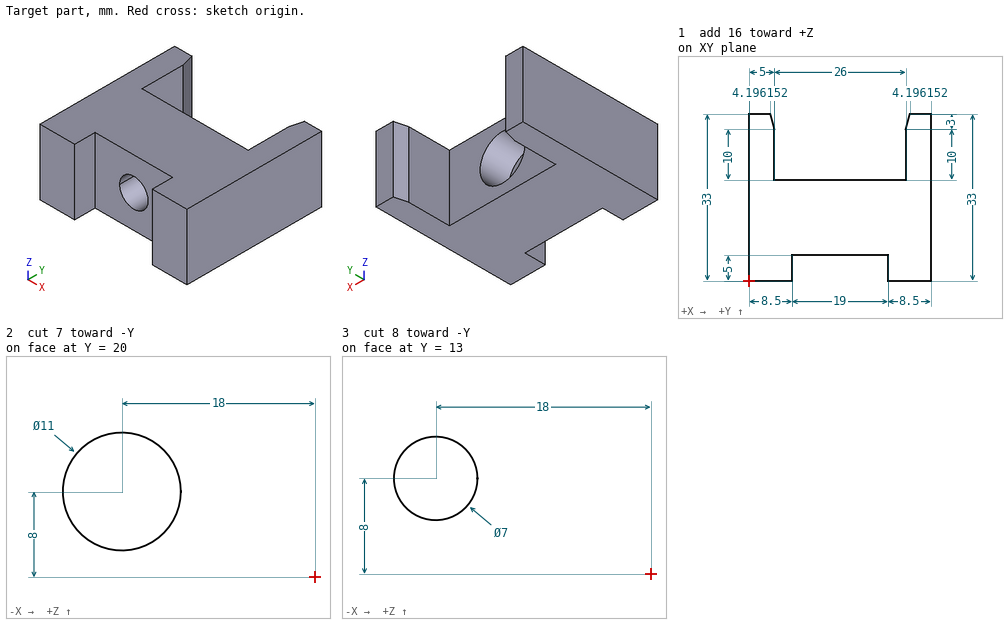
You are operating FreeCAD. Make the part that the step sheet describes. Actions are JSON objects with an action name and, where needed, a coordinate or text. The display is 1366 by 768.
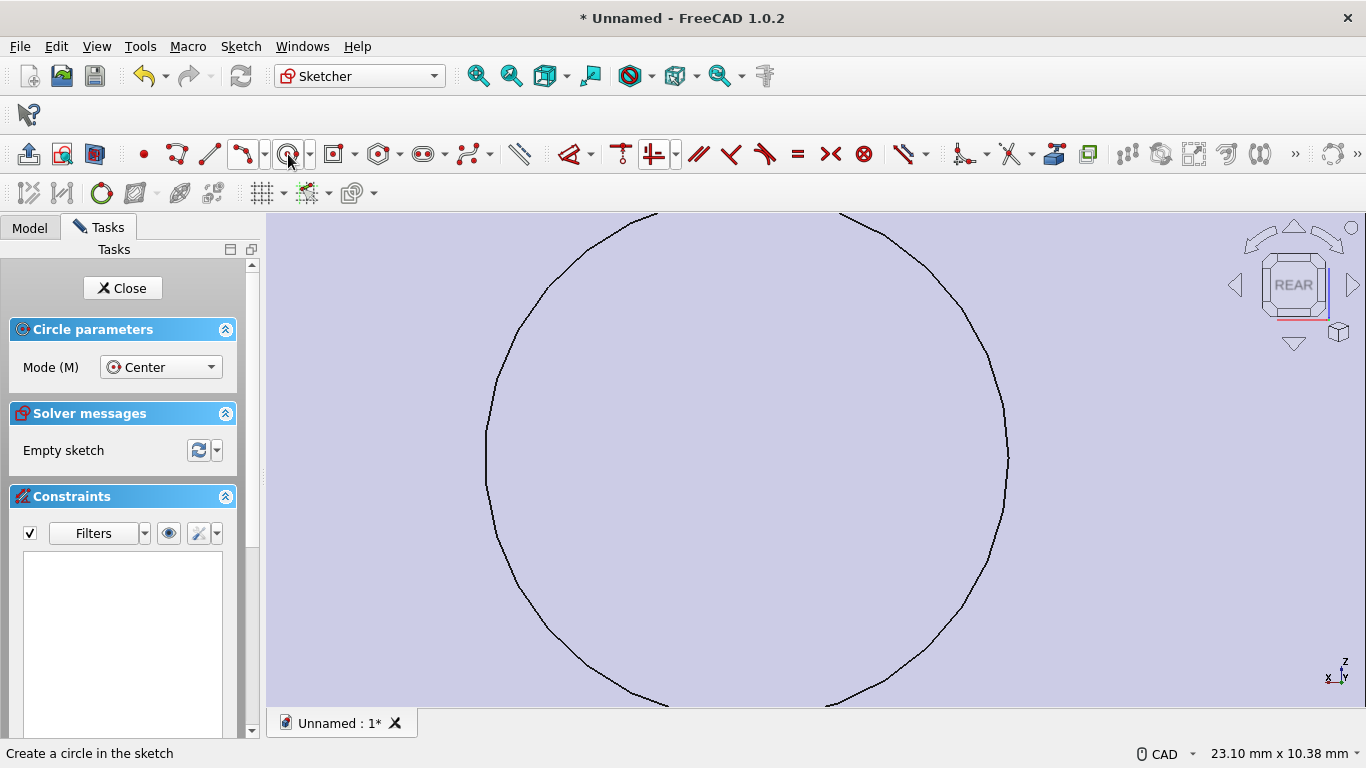
{"action": "left_click", "coordinate": [747, 458]}
{"action": "mouse_move", "coordinate": [865, 340]}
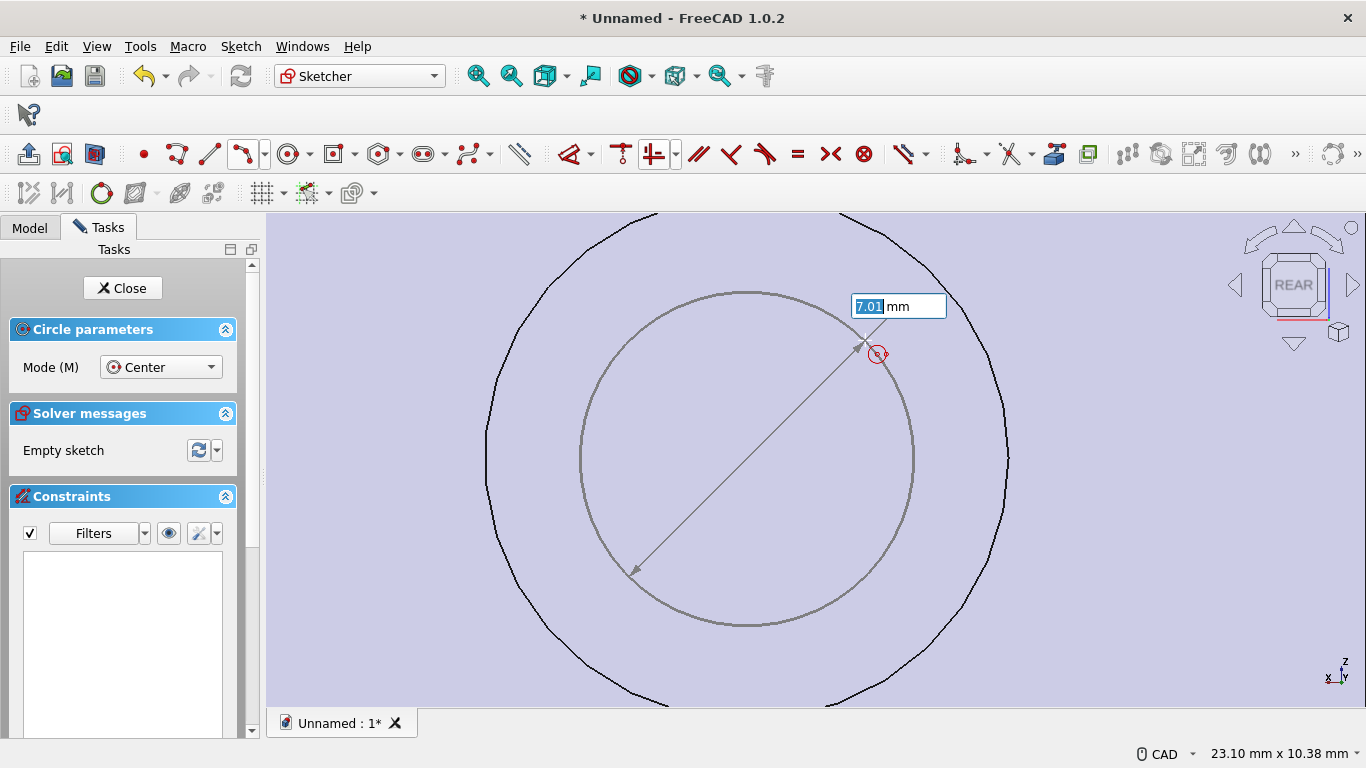
{"action": "type", "text": "7"}
{"action": "key", "text": "Return"}
{"action": "key", "text": "Escape"}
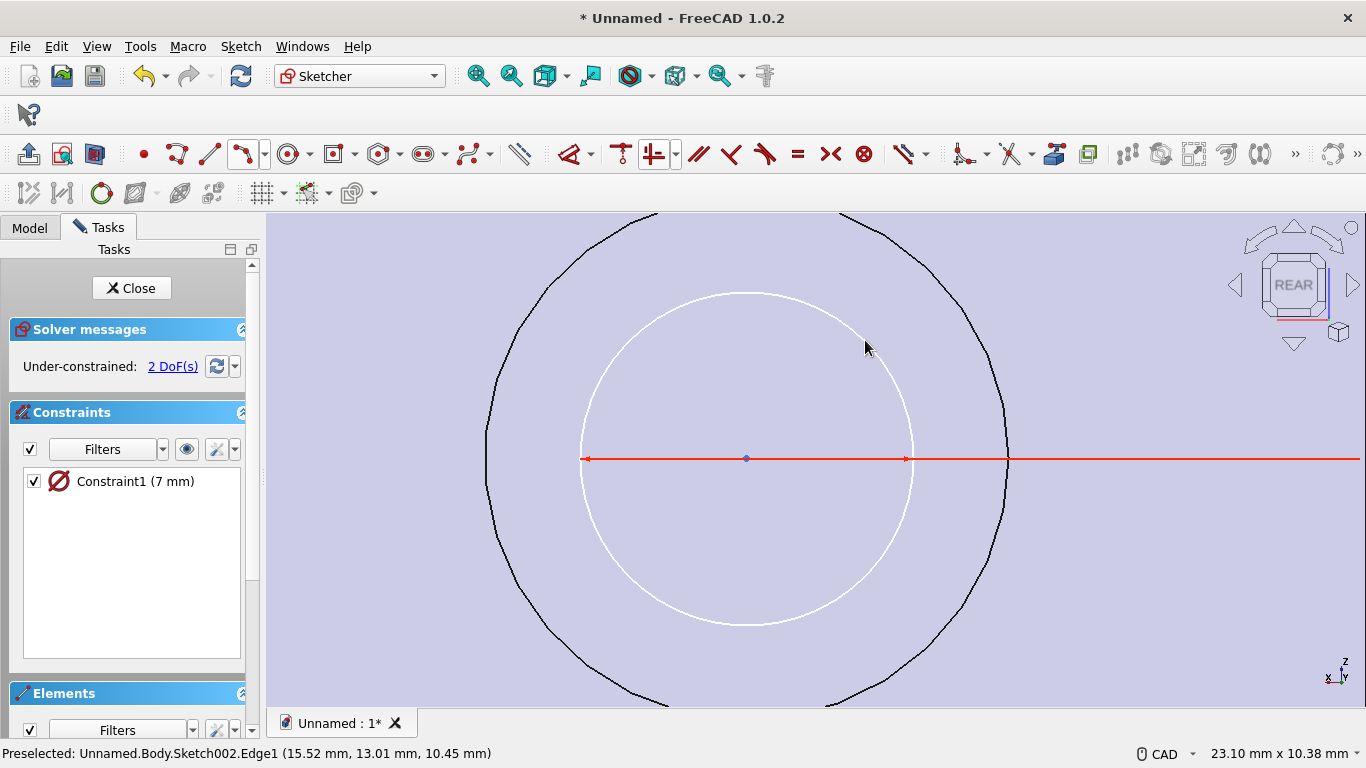
{"action": "left_click", "coordinate": [568, 154]}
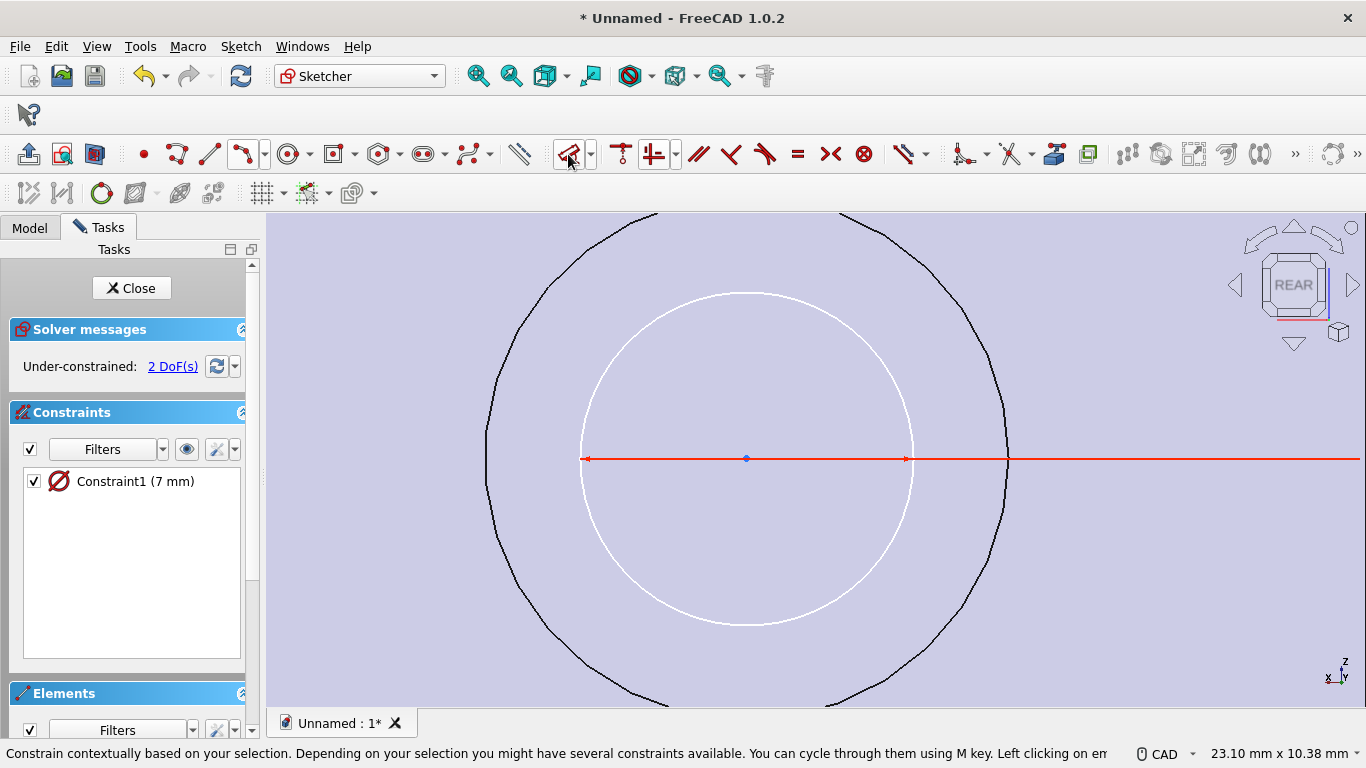
{"action": "left_click", "coordinate": [747, 459]}
{"action": "left_click", "coordinate": [713, 569]}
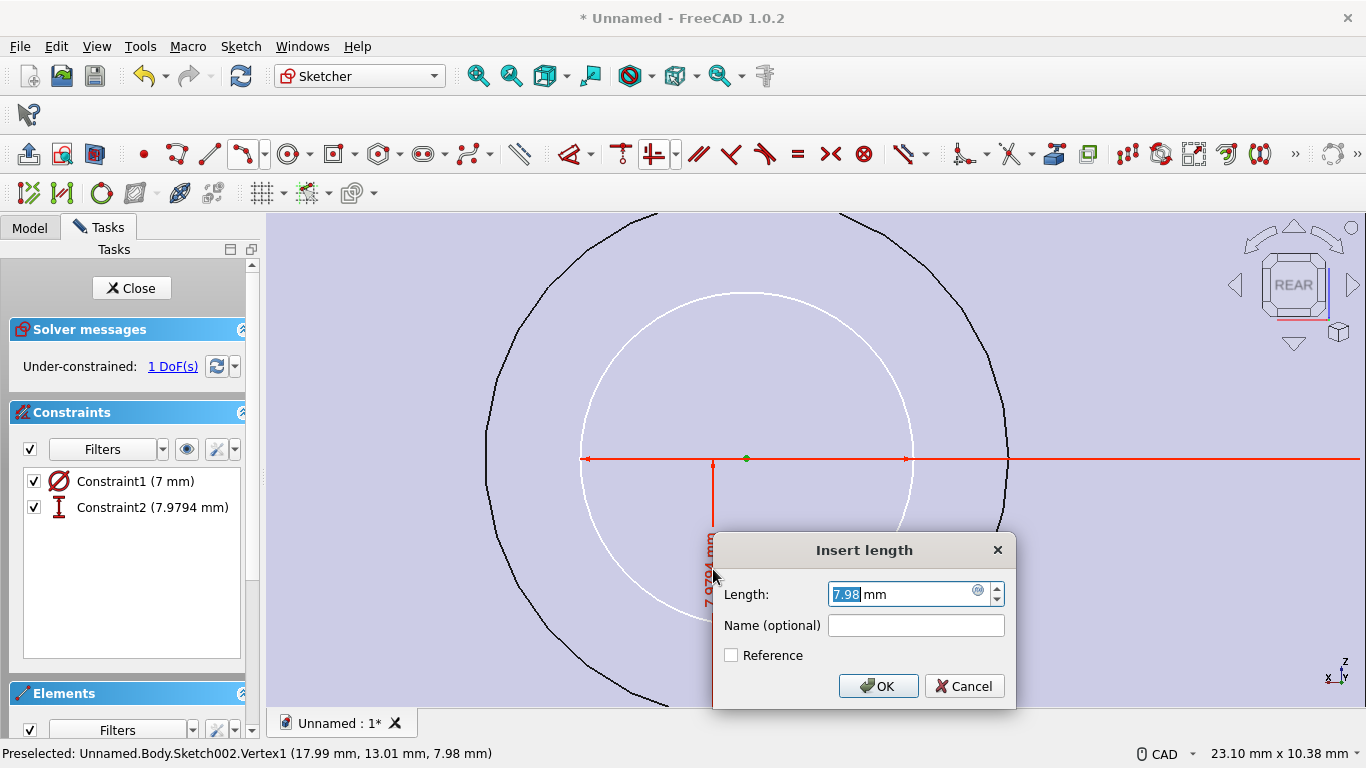
{"action": "type", "text": "8"}
{"action": "key", "text": "Return"}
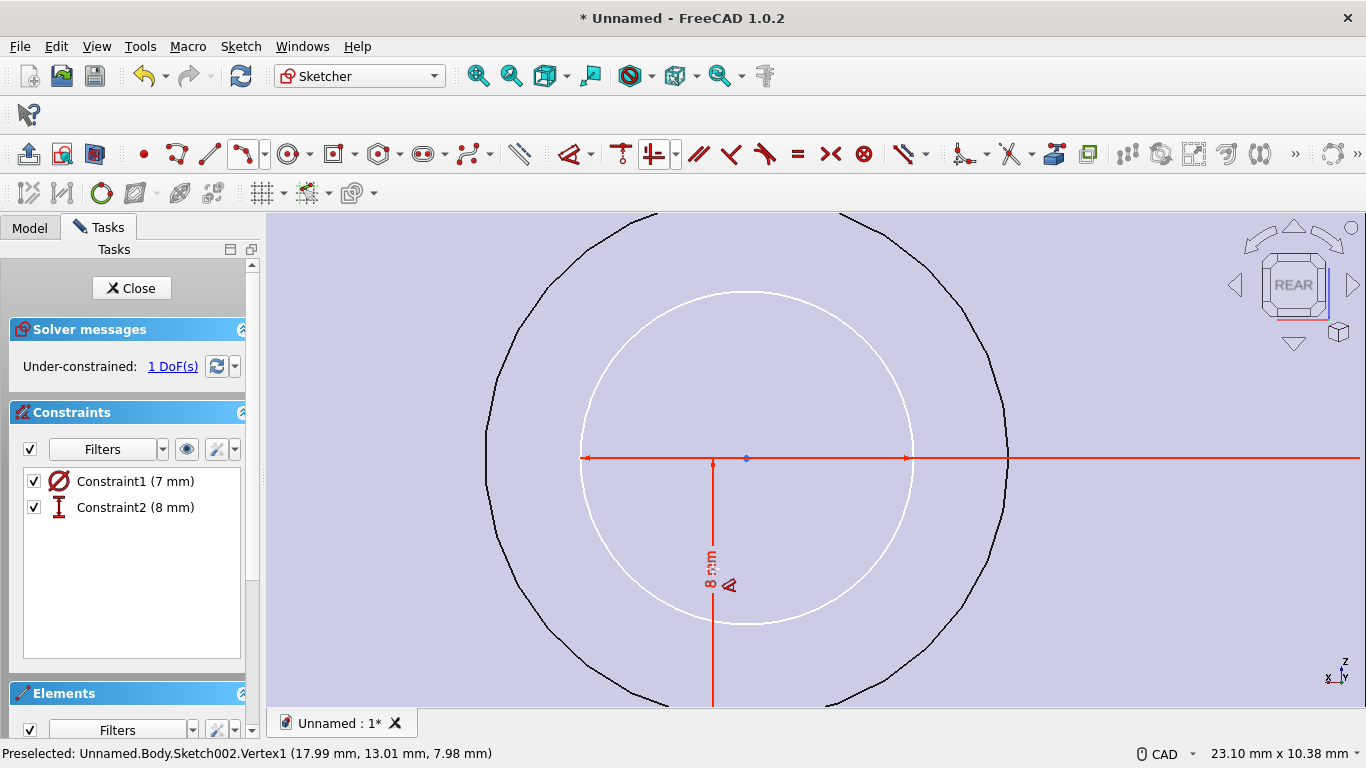
{"action": "left_click", "coordinate": [747, 458]}
{"action": "left_click", "coordinate": [974, 424]}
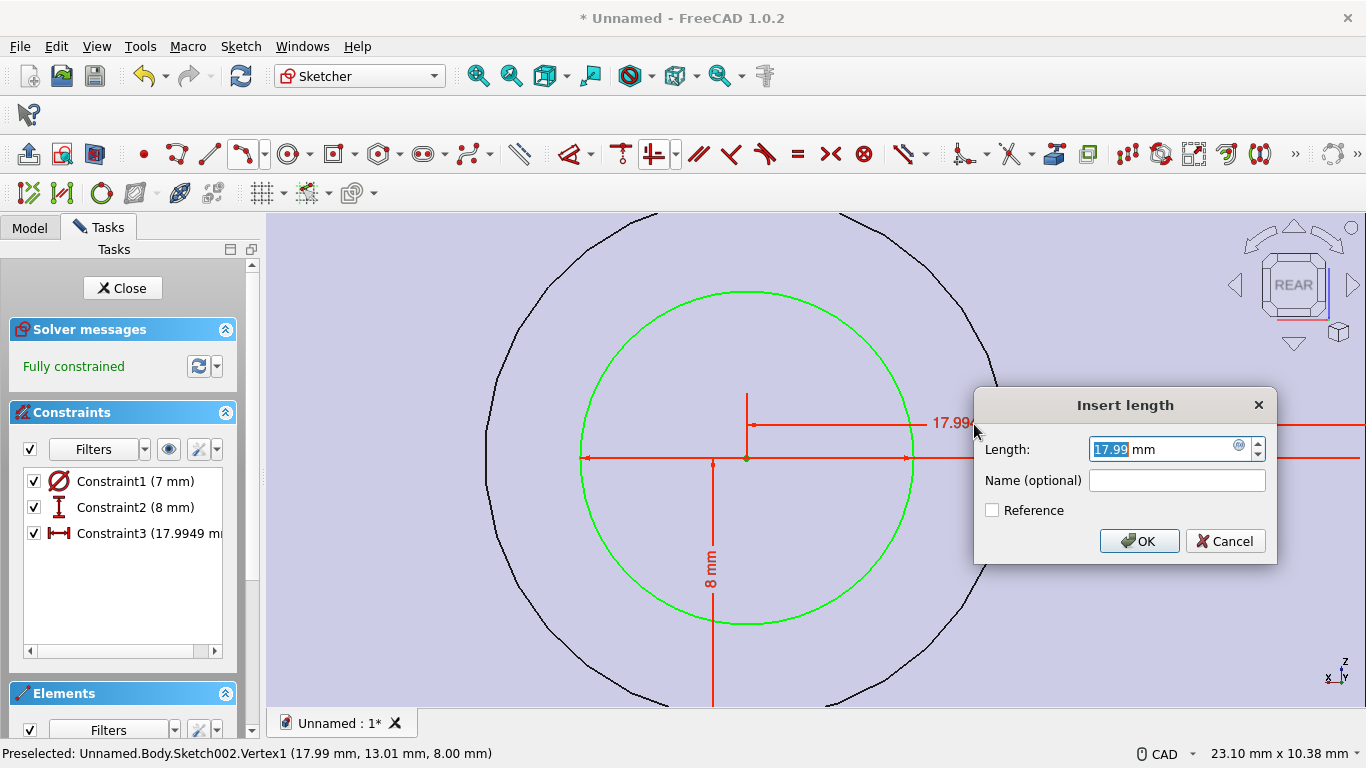
{"action": "type", "text": "18"}
{"action": "key", "text": "Return"}
{"action": "key", "text": "Escape"}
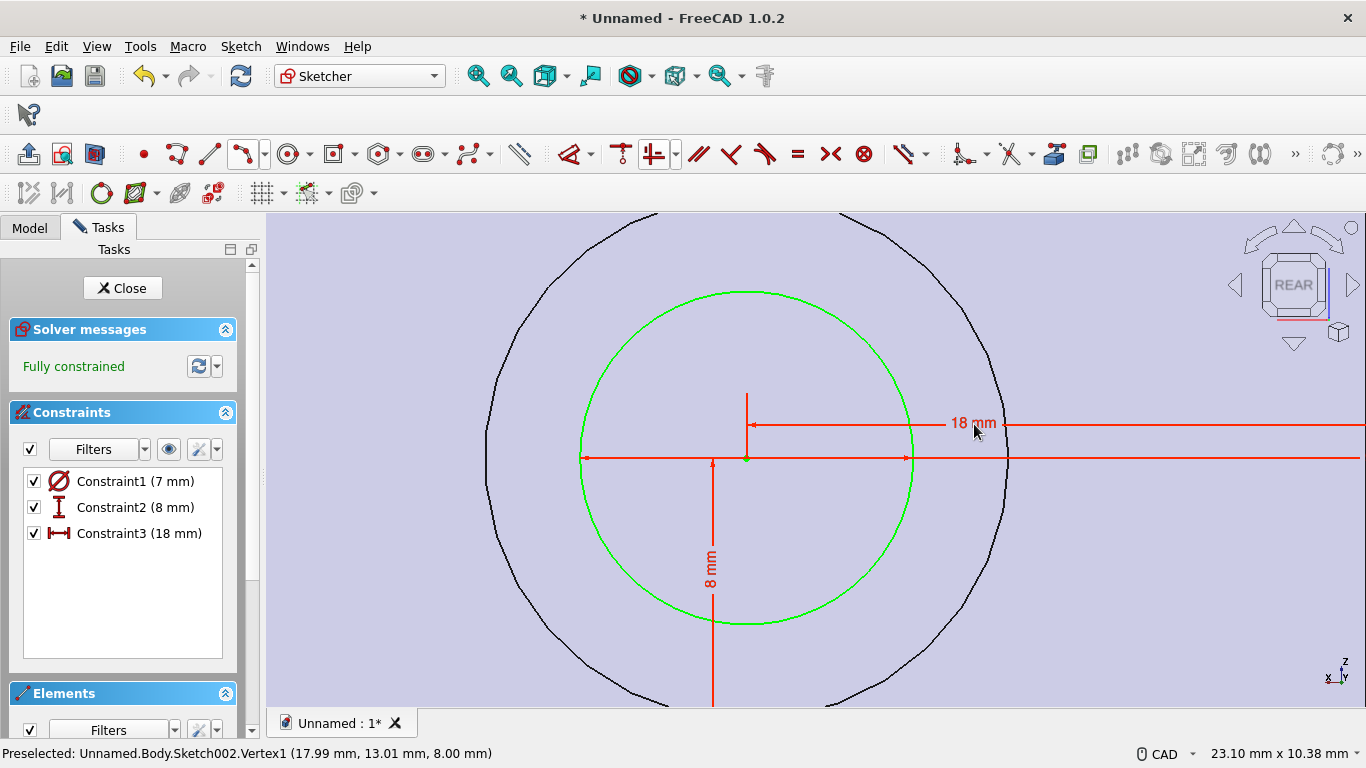
{"action": "left_click", "coordinate": [123, 288]}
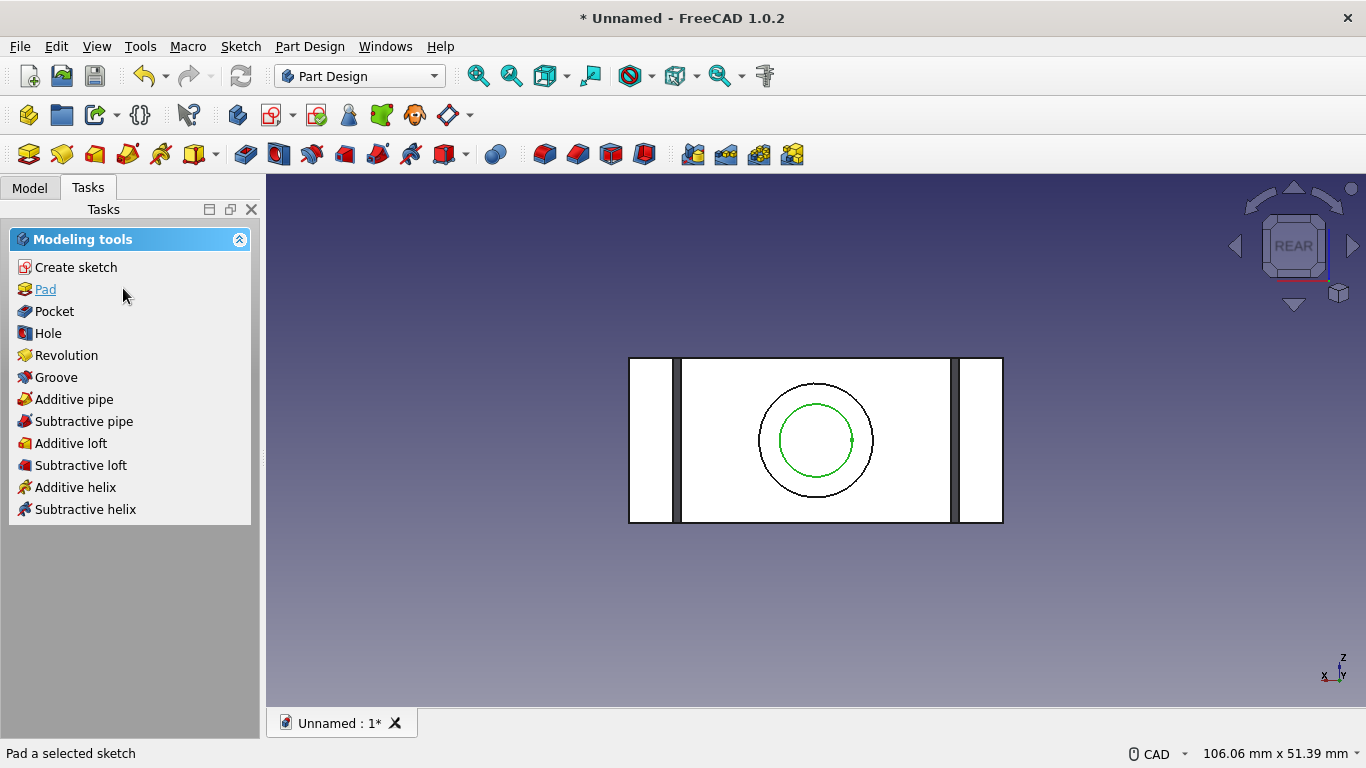
{"action": "left_click", "coordinate": [246, 154]}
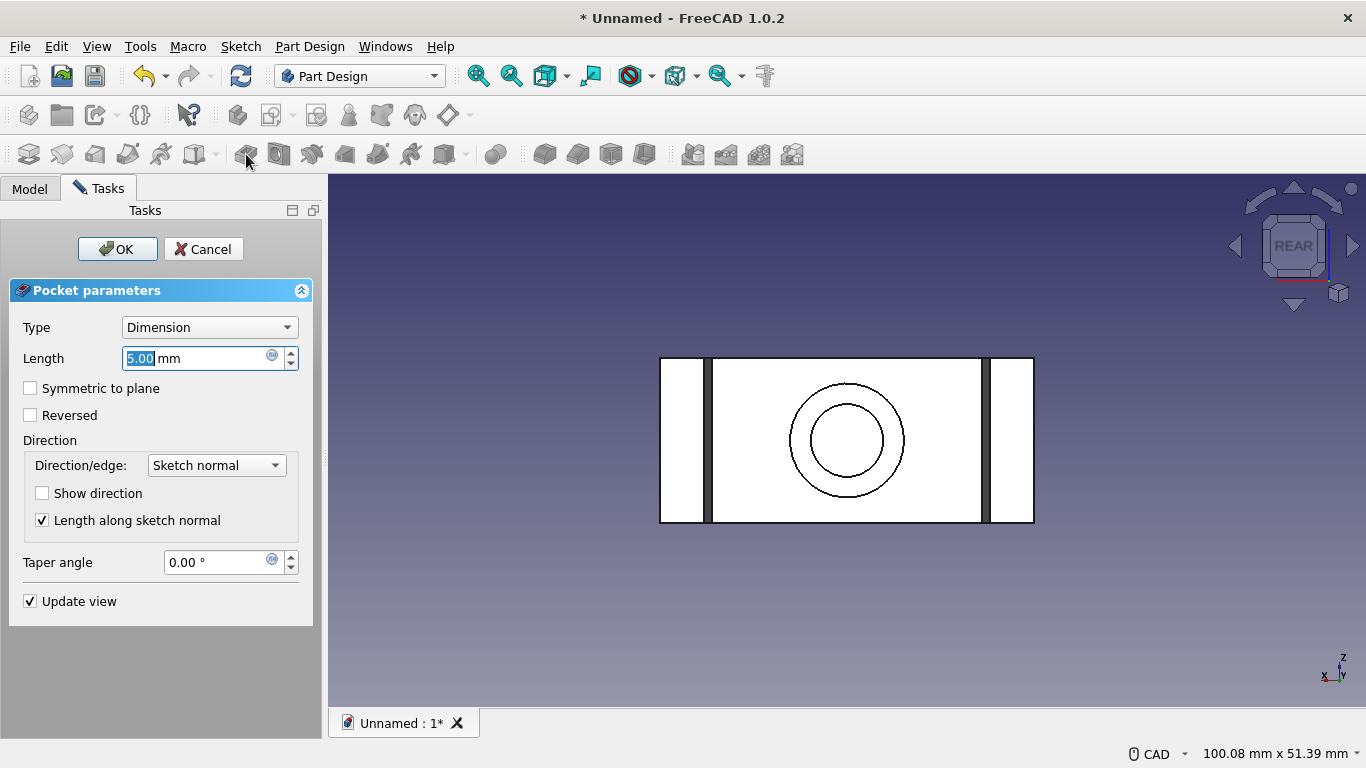
{"action": "type", "text": "8"}
{"action": "key", "text": "Tab"}